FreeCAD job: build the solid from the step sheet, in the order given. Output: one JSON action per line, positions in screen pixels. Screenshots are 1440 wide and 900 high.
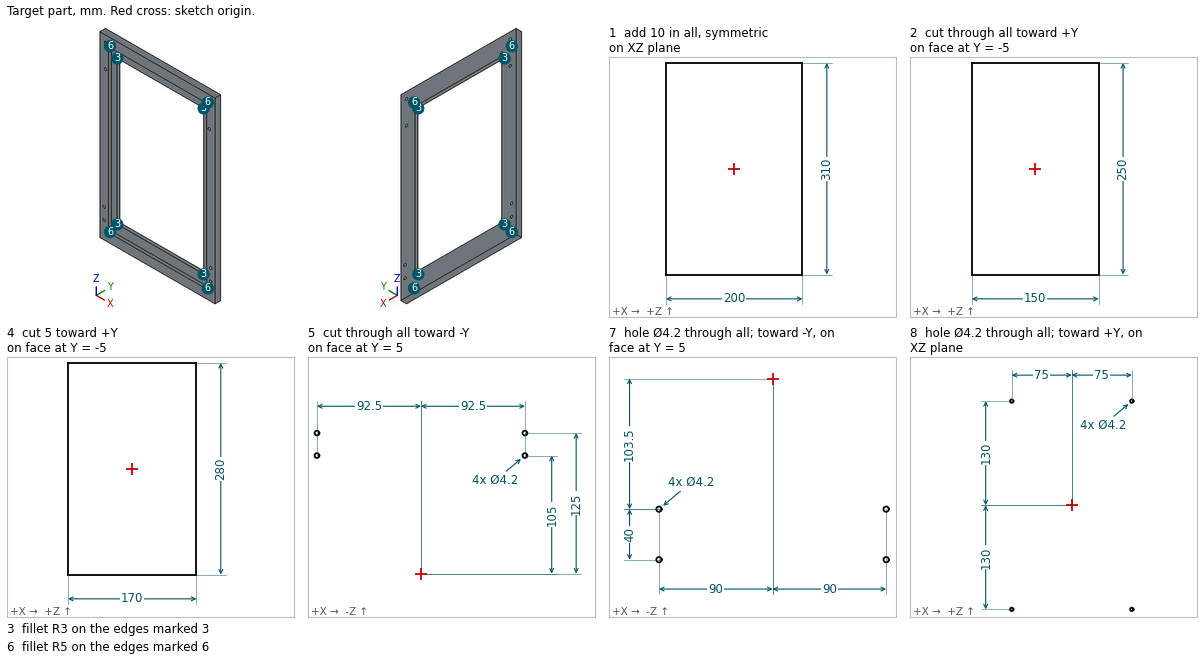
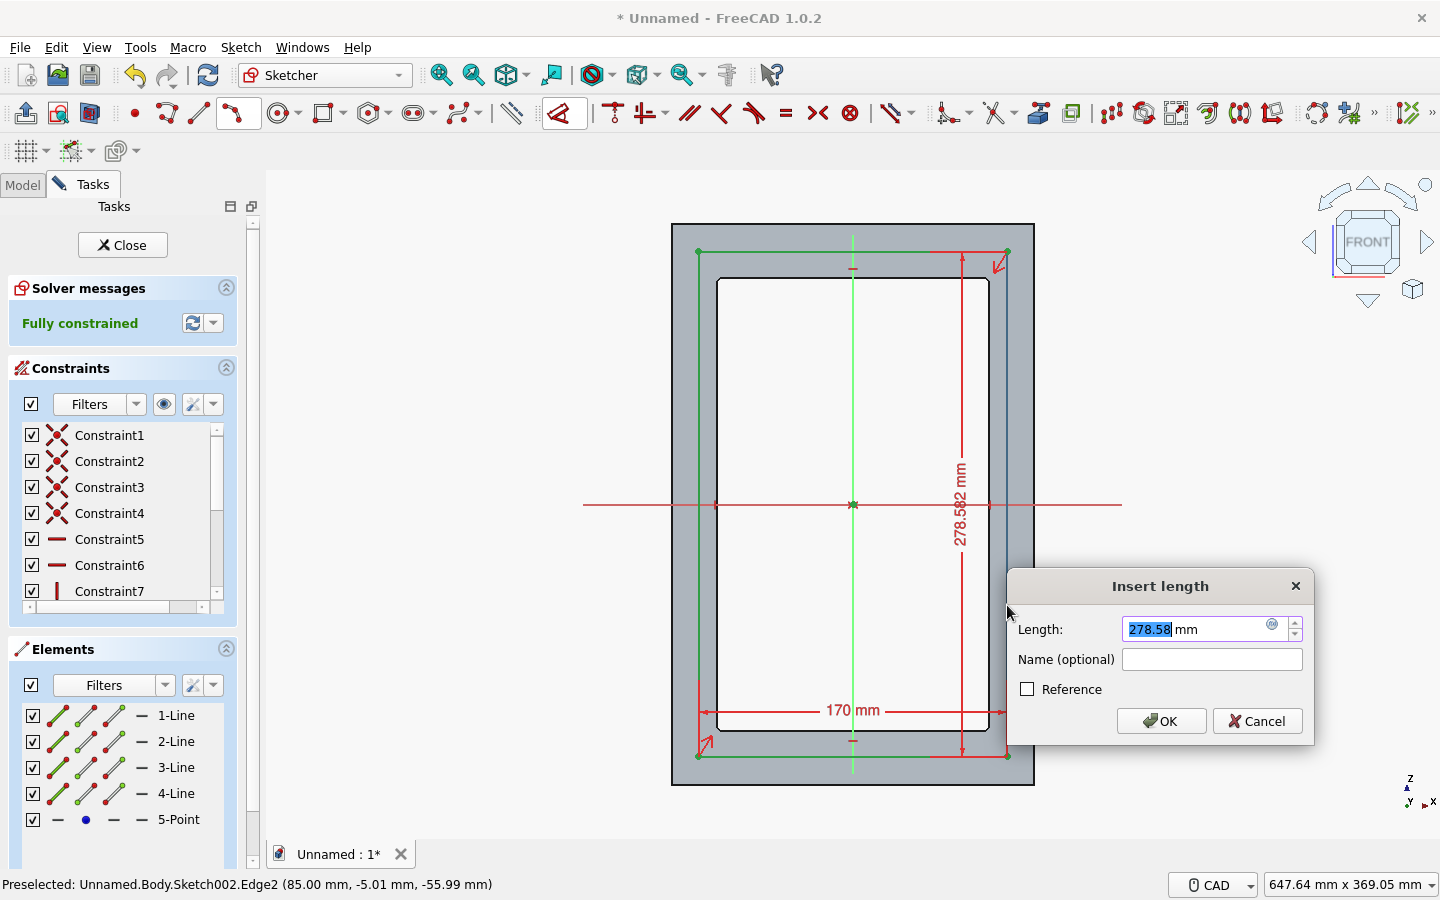
{"action": "type", "text": "280"}
{"action": "key", "text": "Return"}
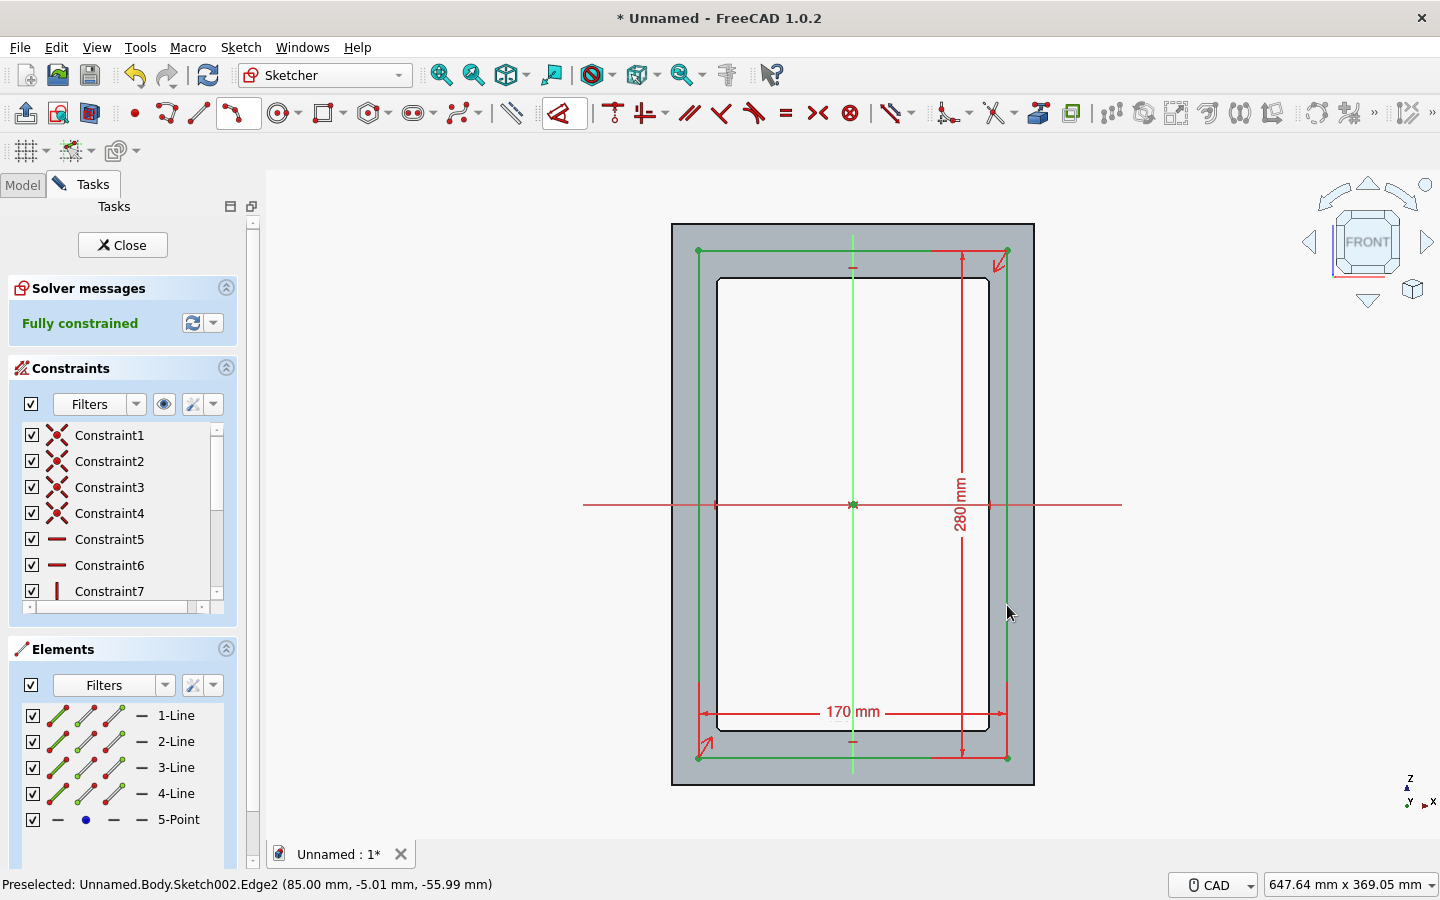
{"action": "left_click", "coordinate": [123, 245]}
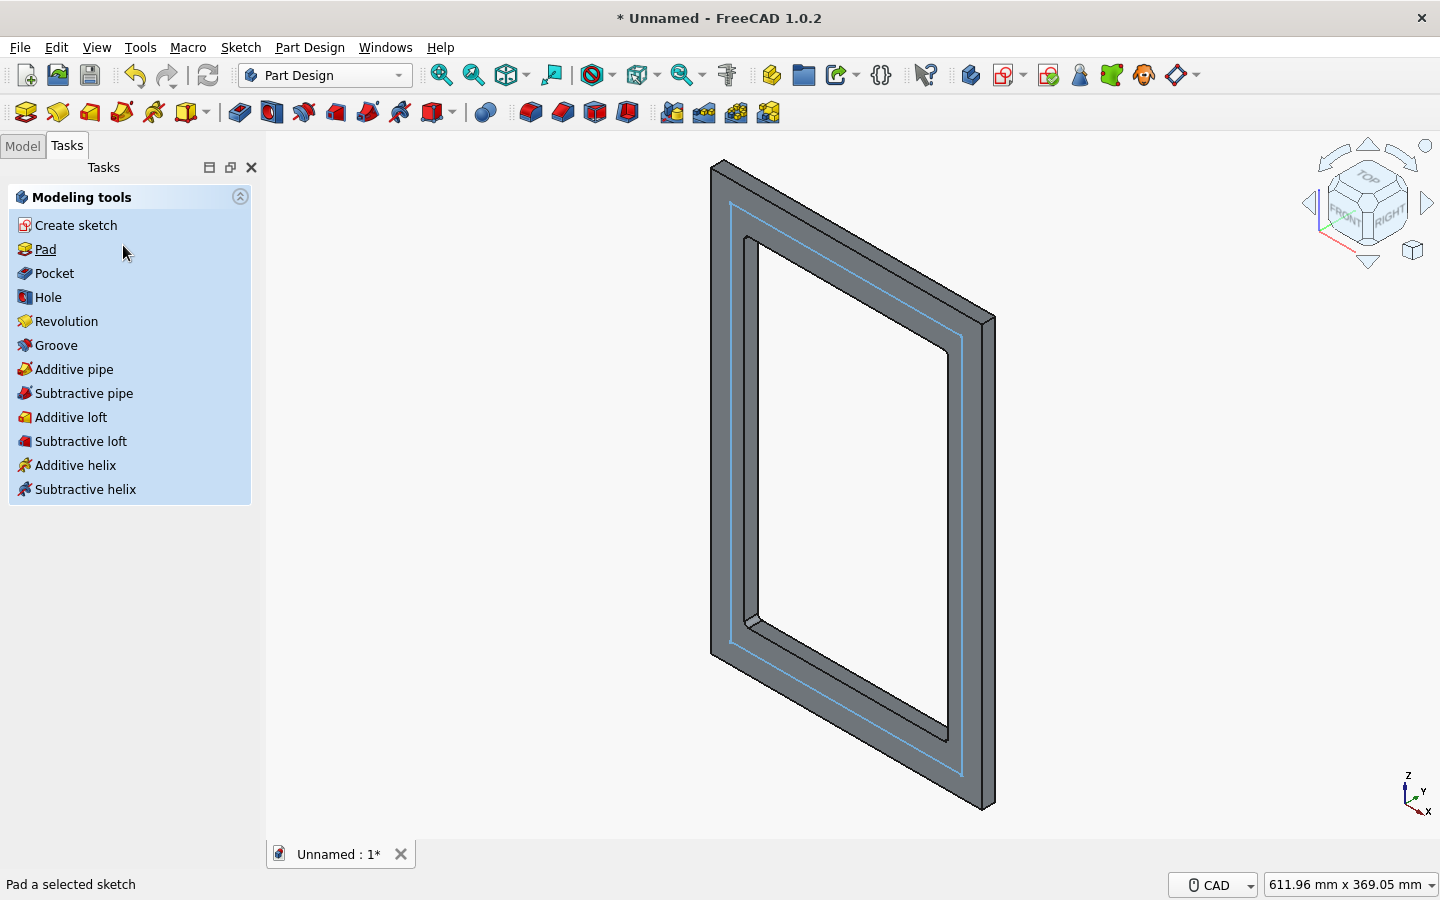
{"action": "left_click", "coordinate": [240, 112]}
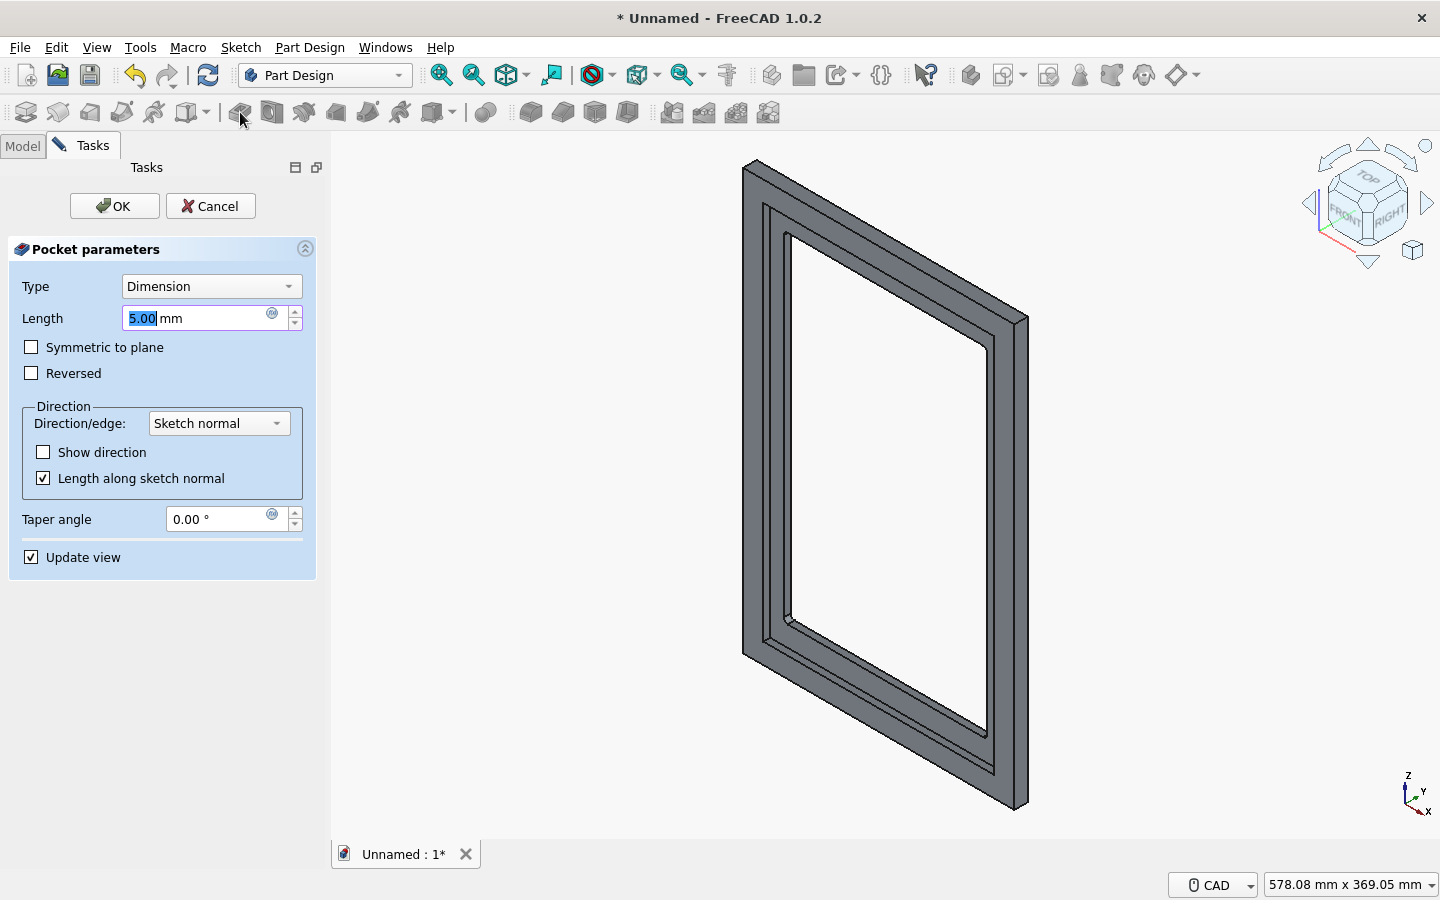
{"action": "type", "text": "5"}
{"action": "key", "text": "Tab"}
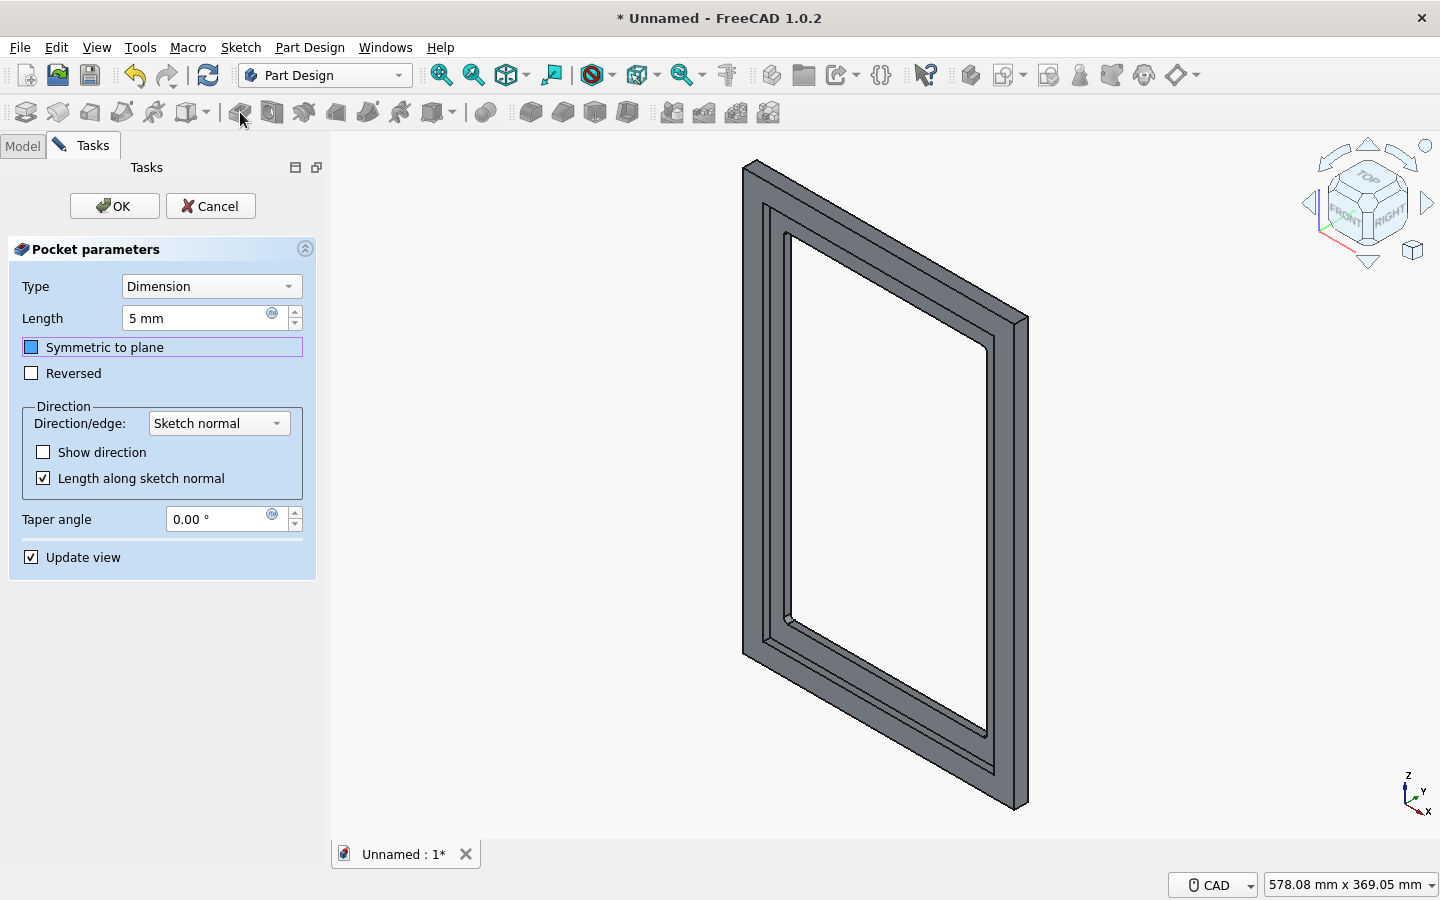
{"action": "left_click", "coordinate": [115, 206]}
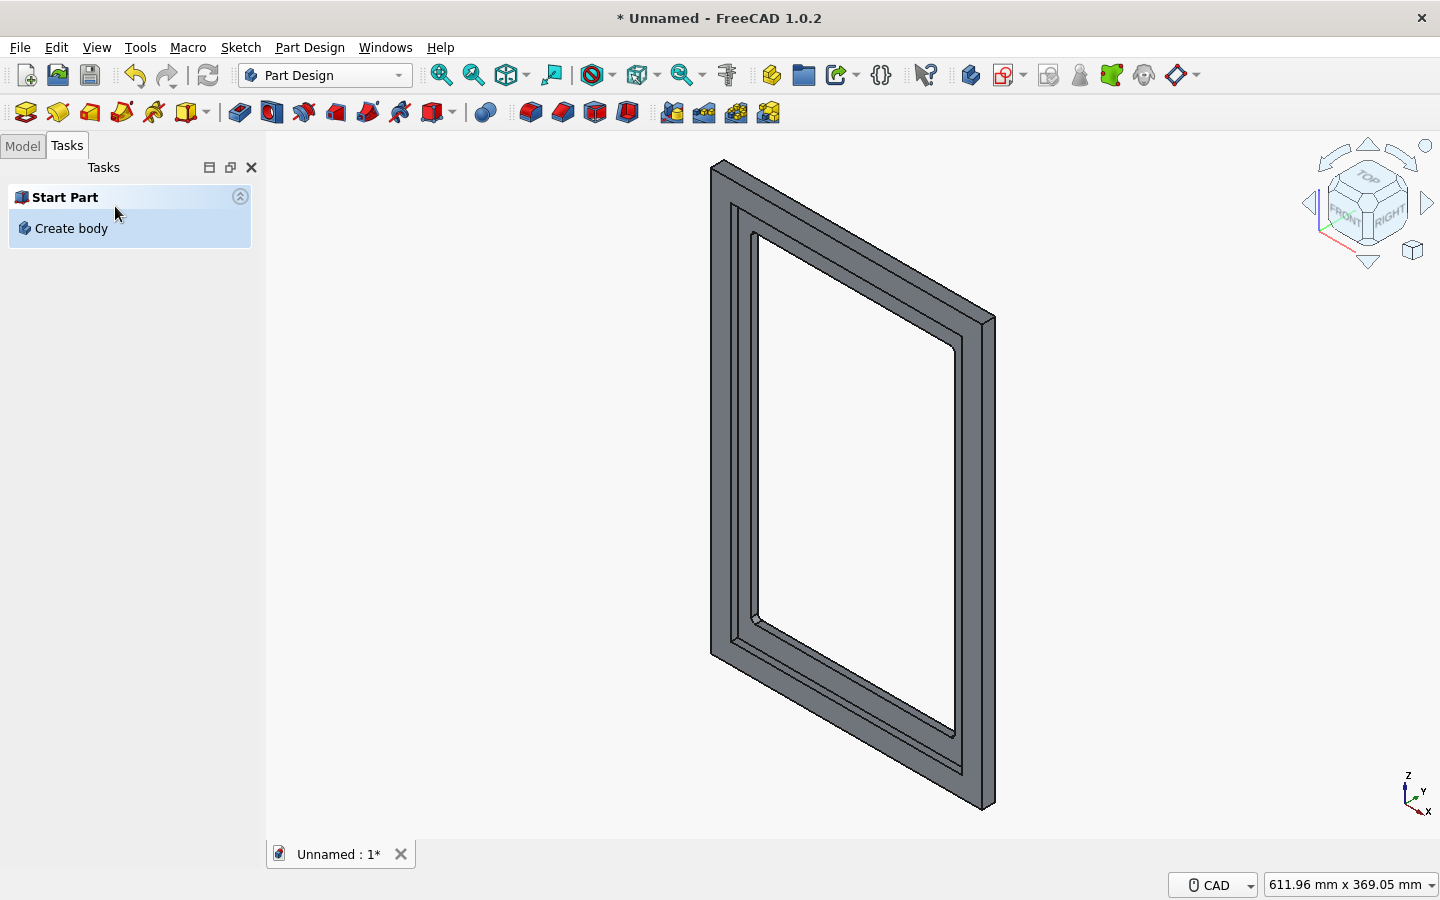
{"action": "key", "text": "4"}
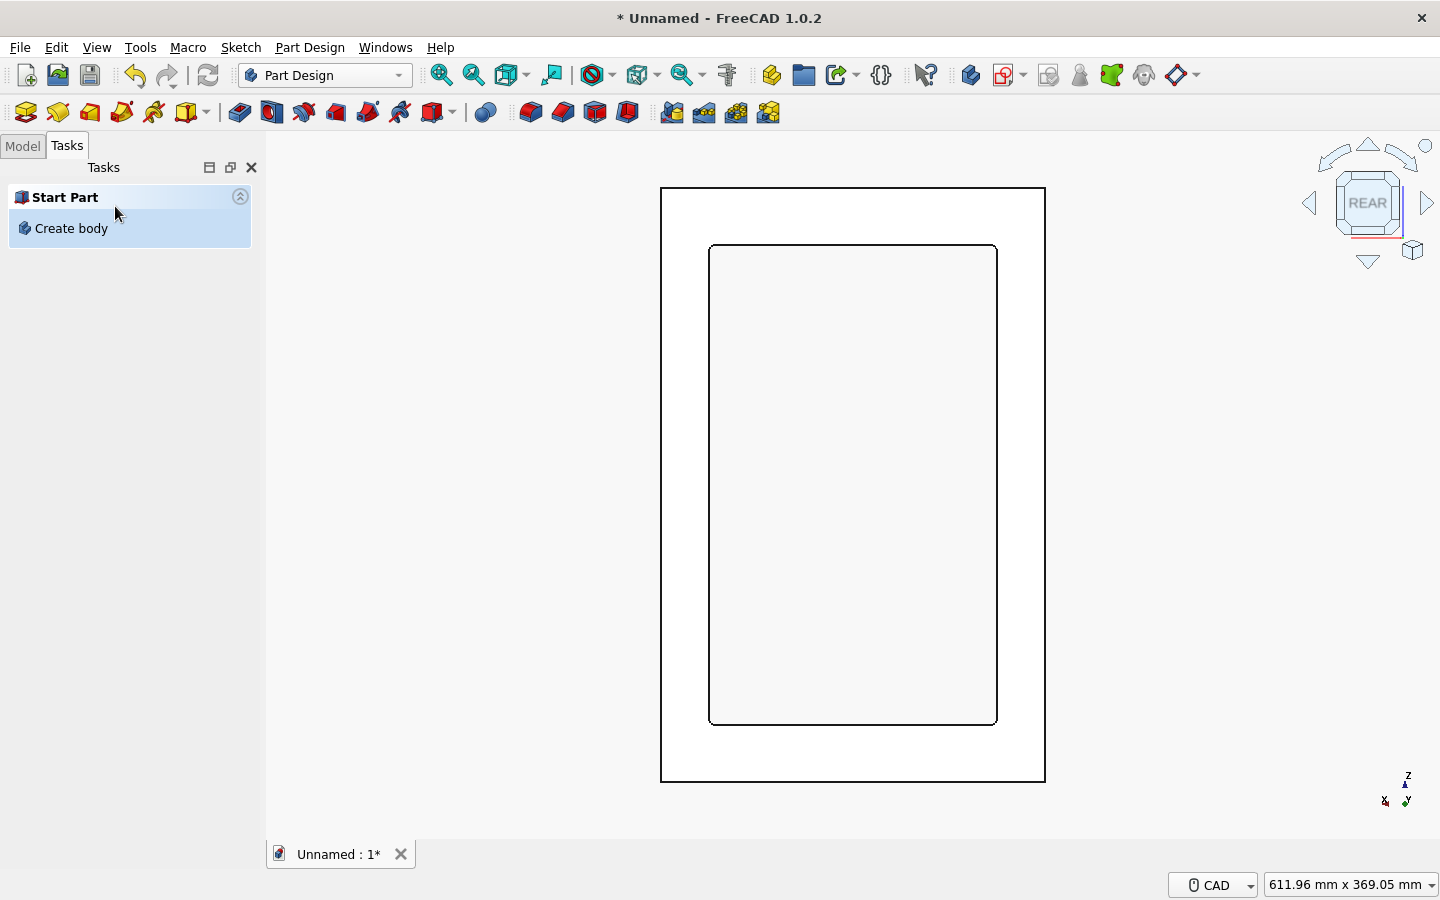
{"action": "left_click", "coordinate": [1017, 229]}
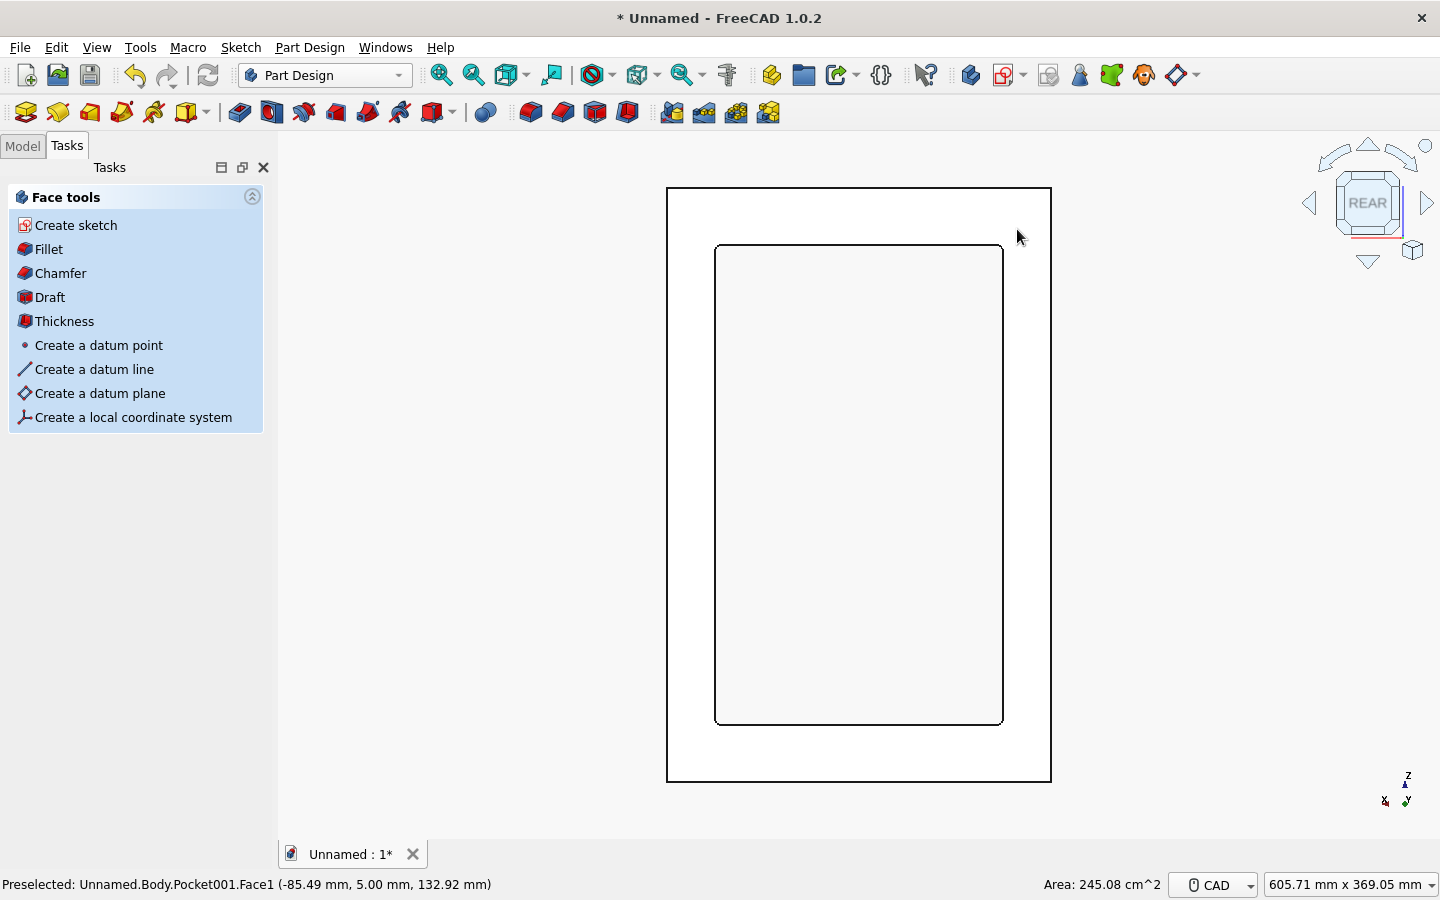
{"action": "left_click", "coordinate": [1004, 76]}